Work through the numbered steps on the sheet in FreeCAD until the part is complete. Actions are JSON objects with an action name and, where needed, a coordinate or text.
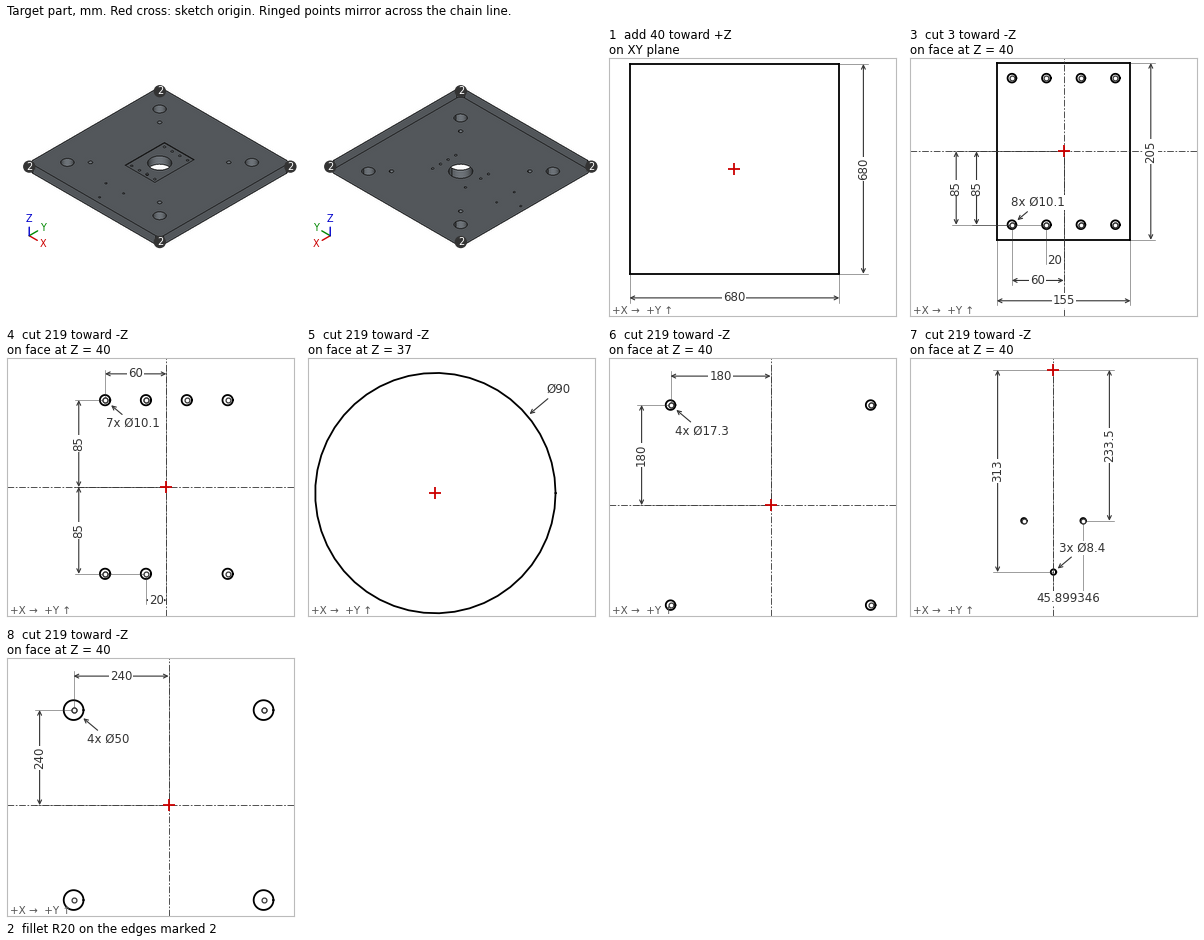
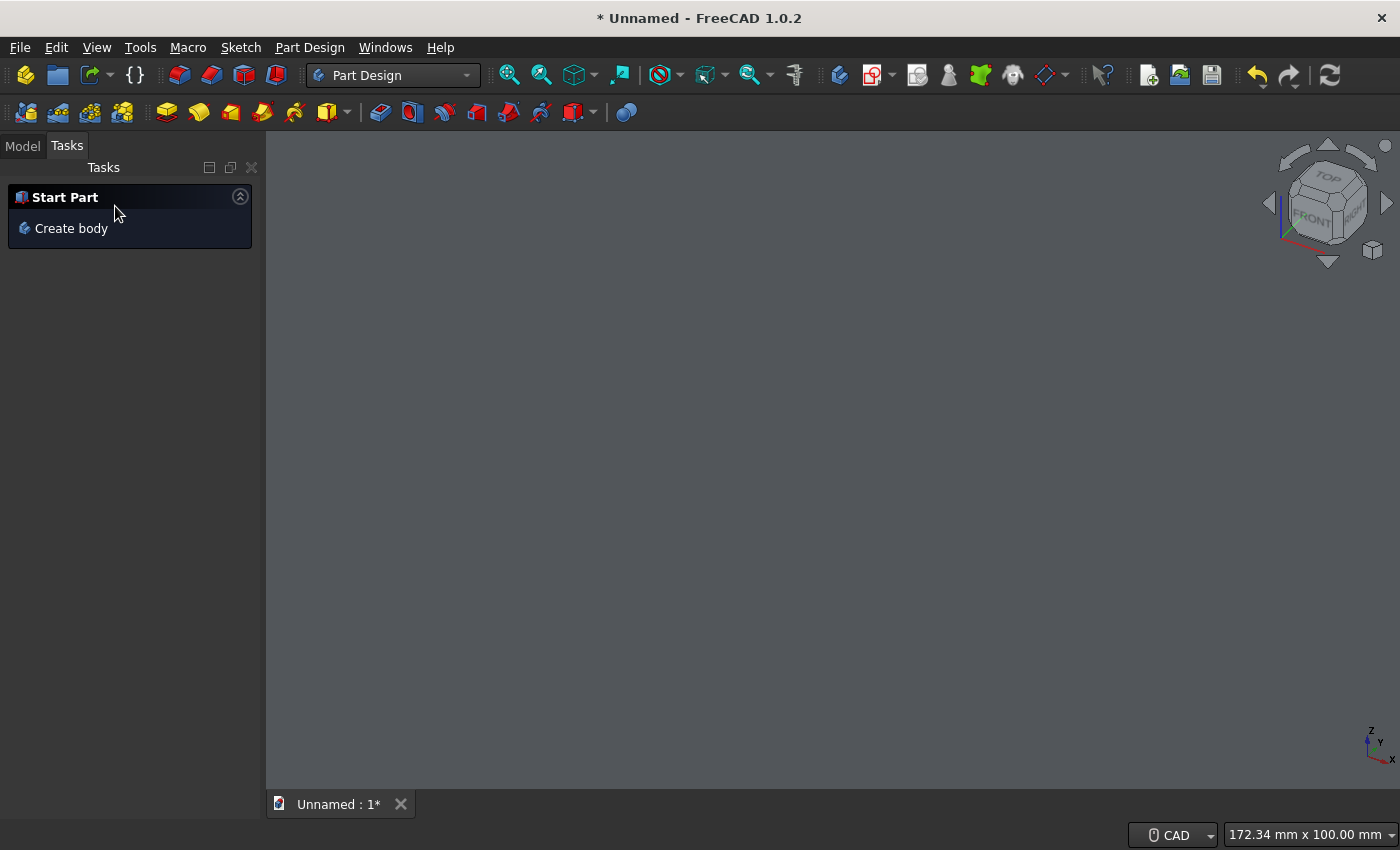
{"action": "left_click", "coordinate": [510, 76]}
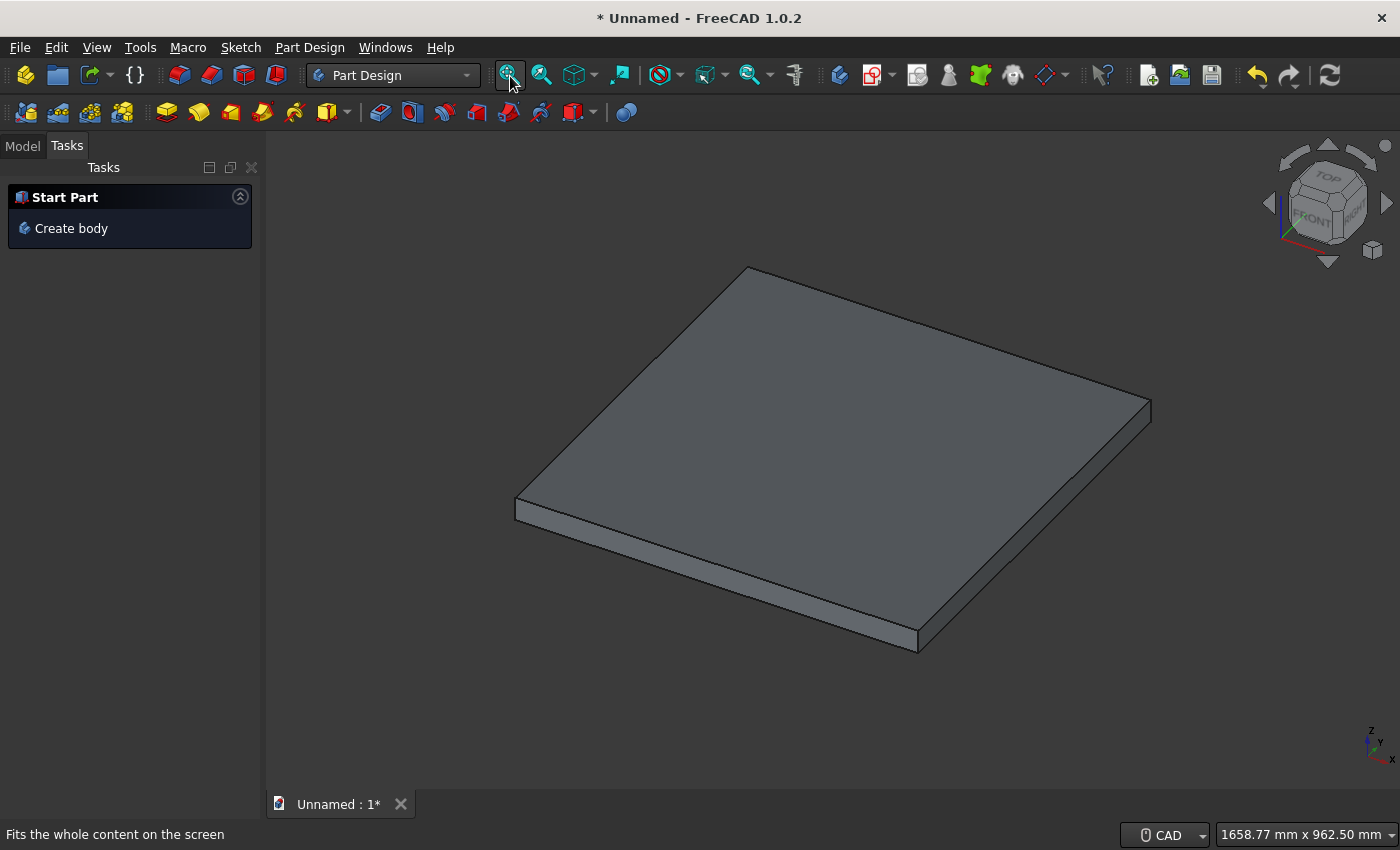
{"action": "left_click", "coordinate": [918, 641]}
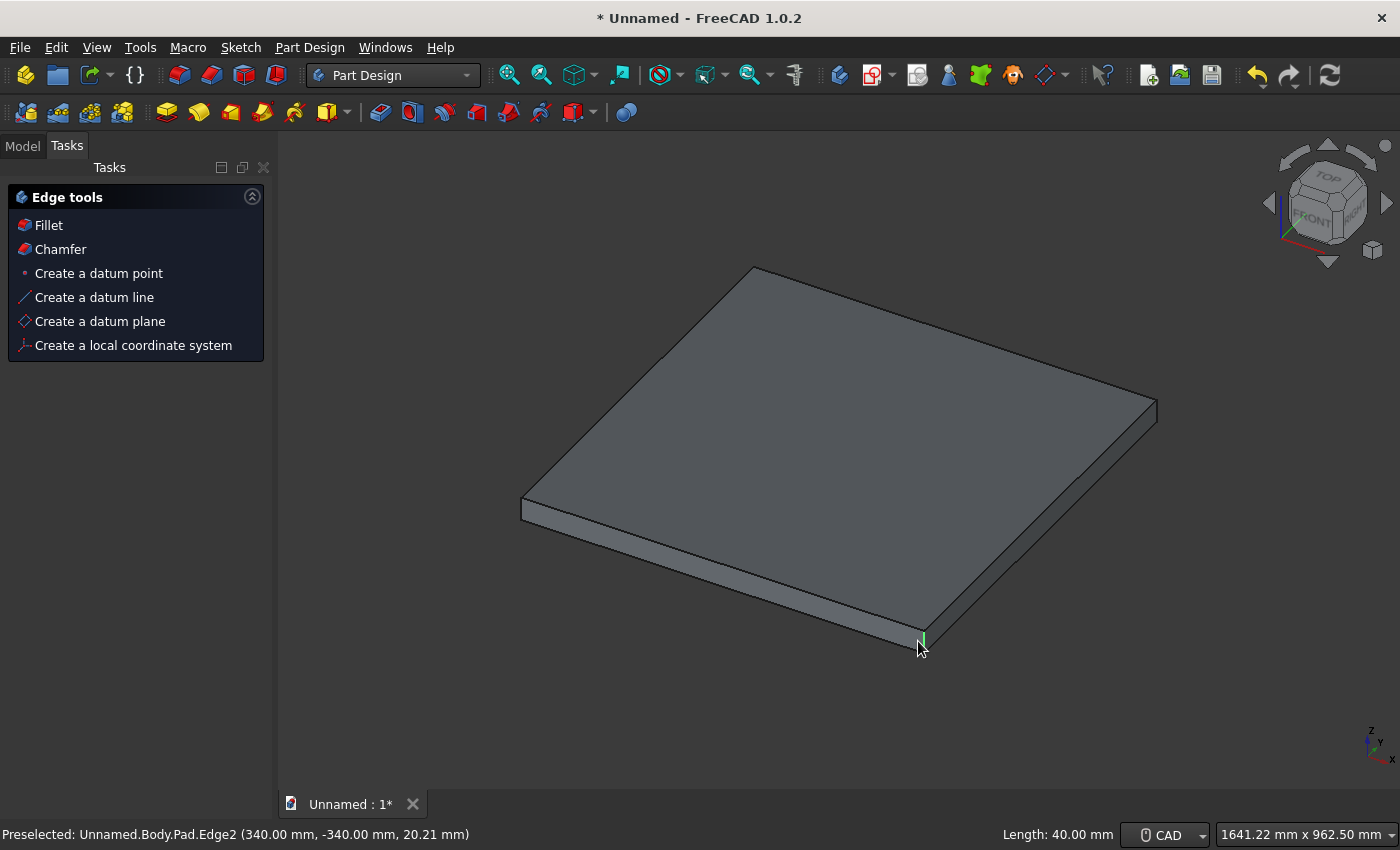
{"action": "key", "text": "0"}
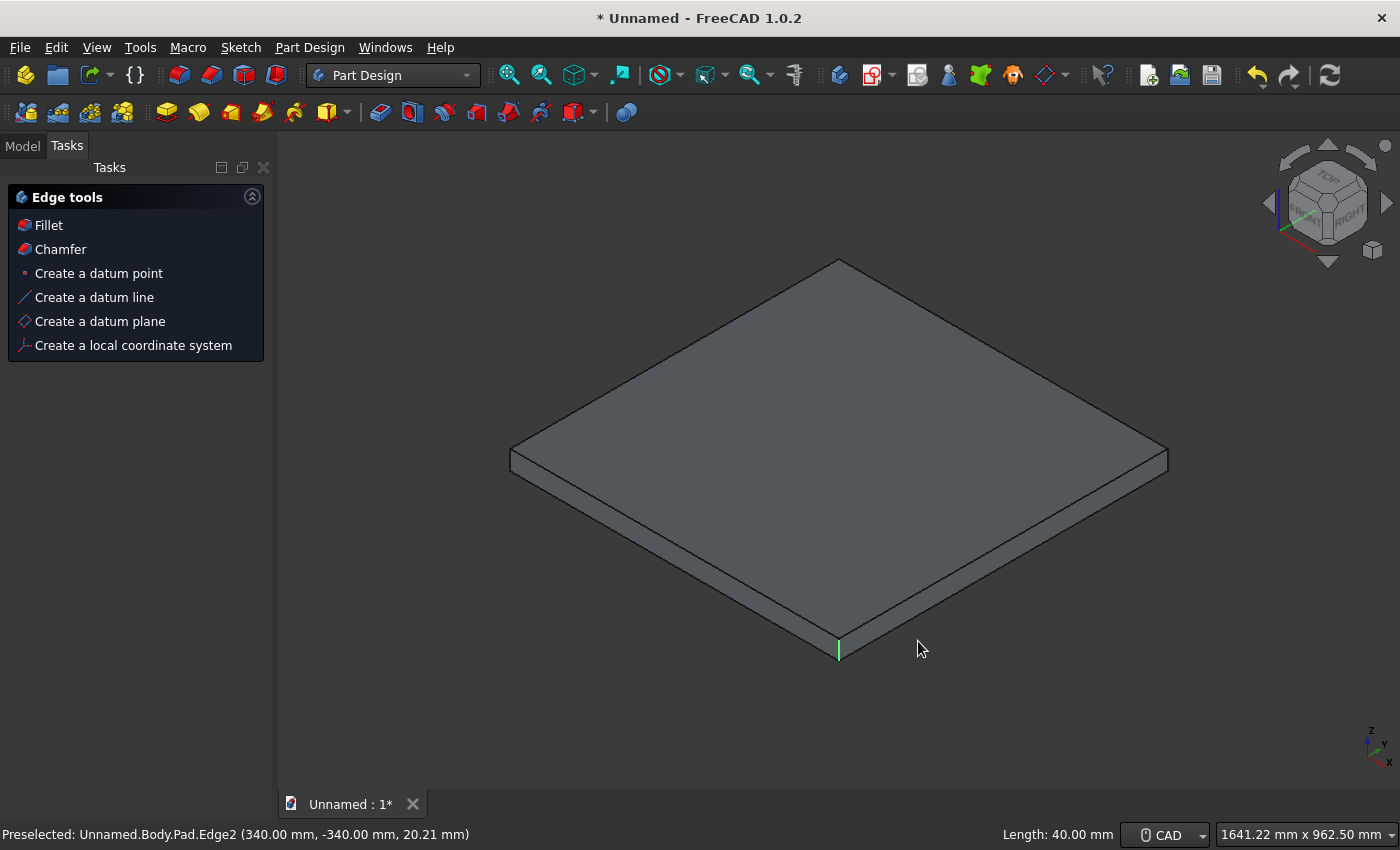
{"action": "key", "text": "2"}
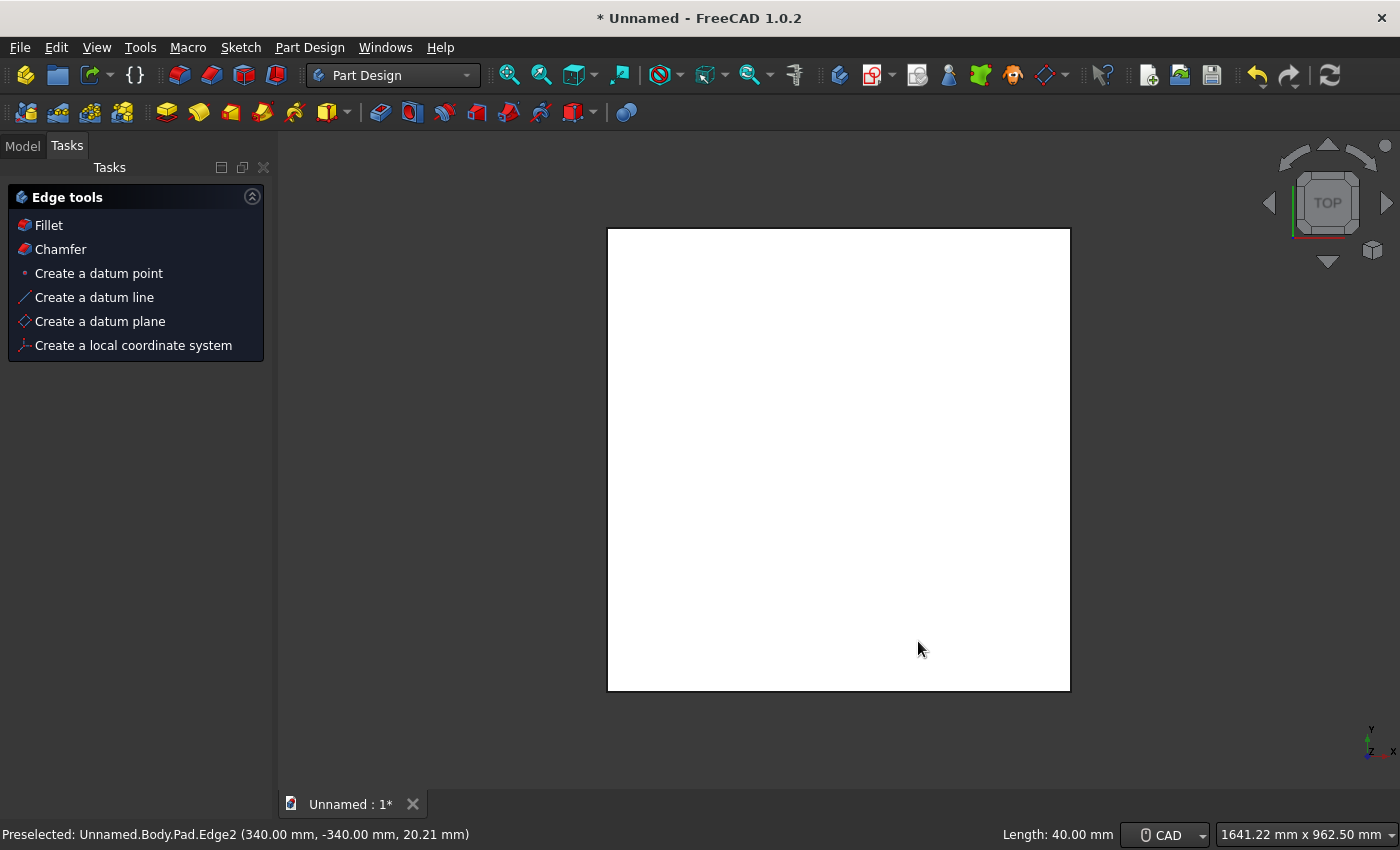
{"action": "key", "text": "1"}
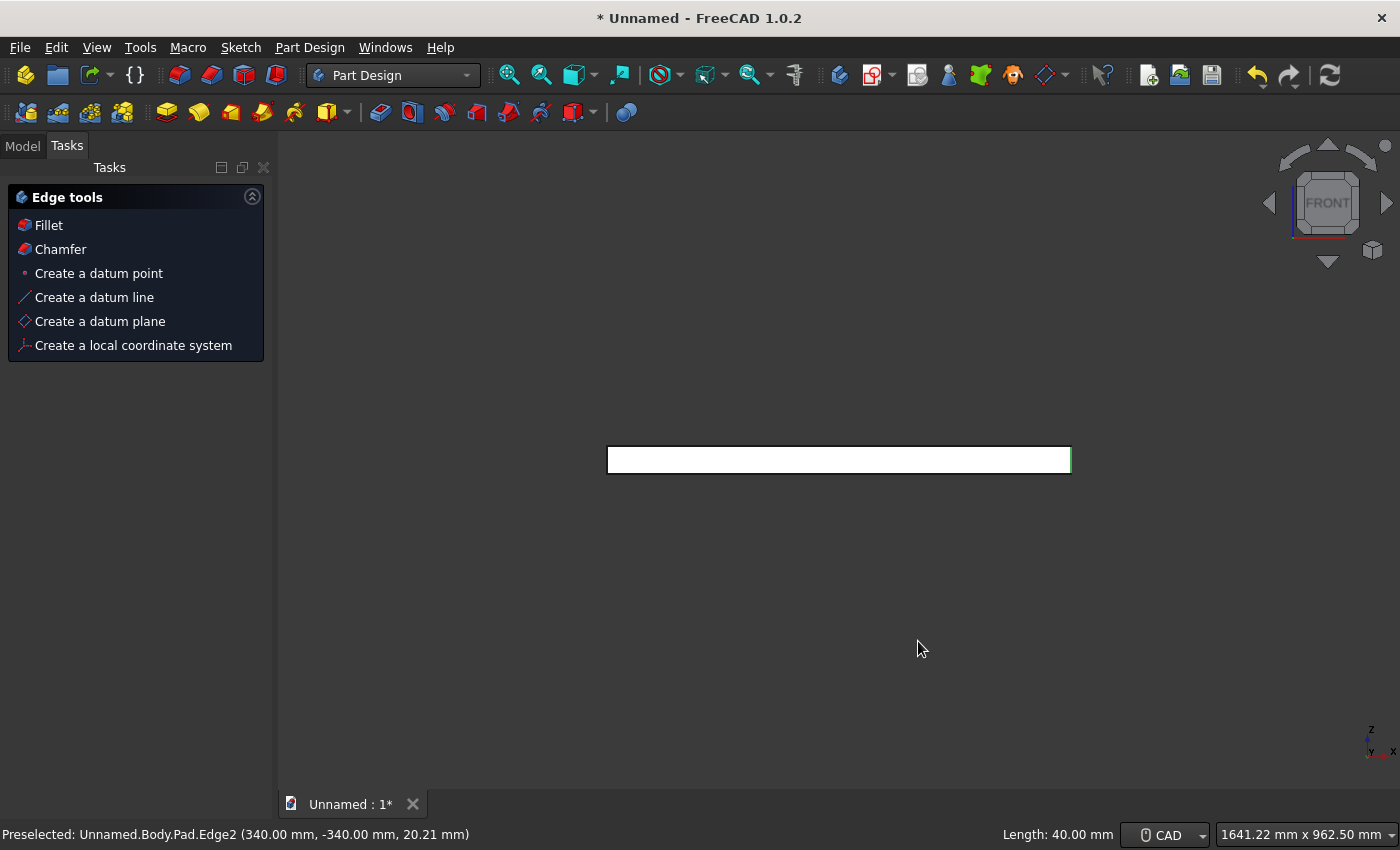
{"action": "left_click", "coordinate": [510, 76]}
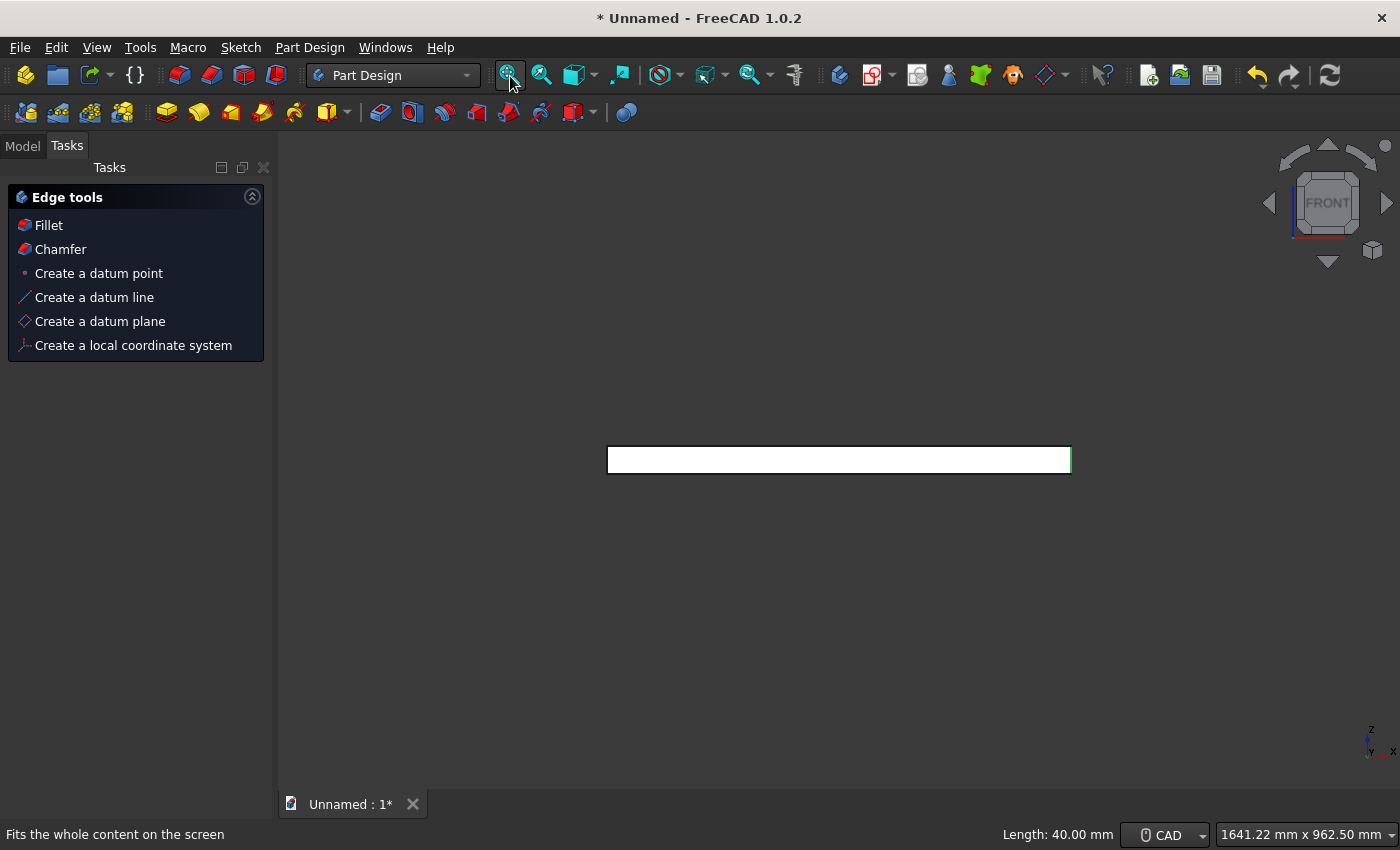
{"action": "left_click", "coordinate": [607, 459], "text": "ctrl"}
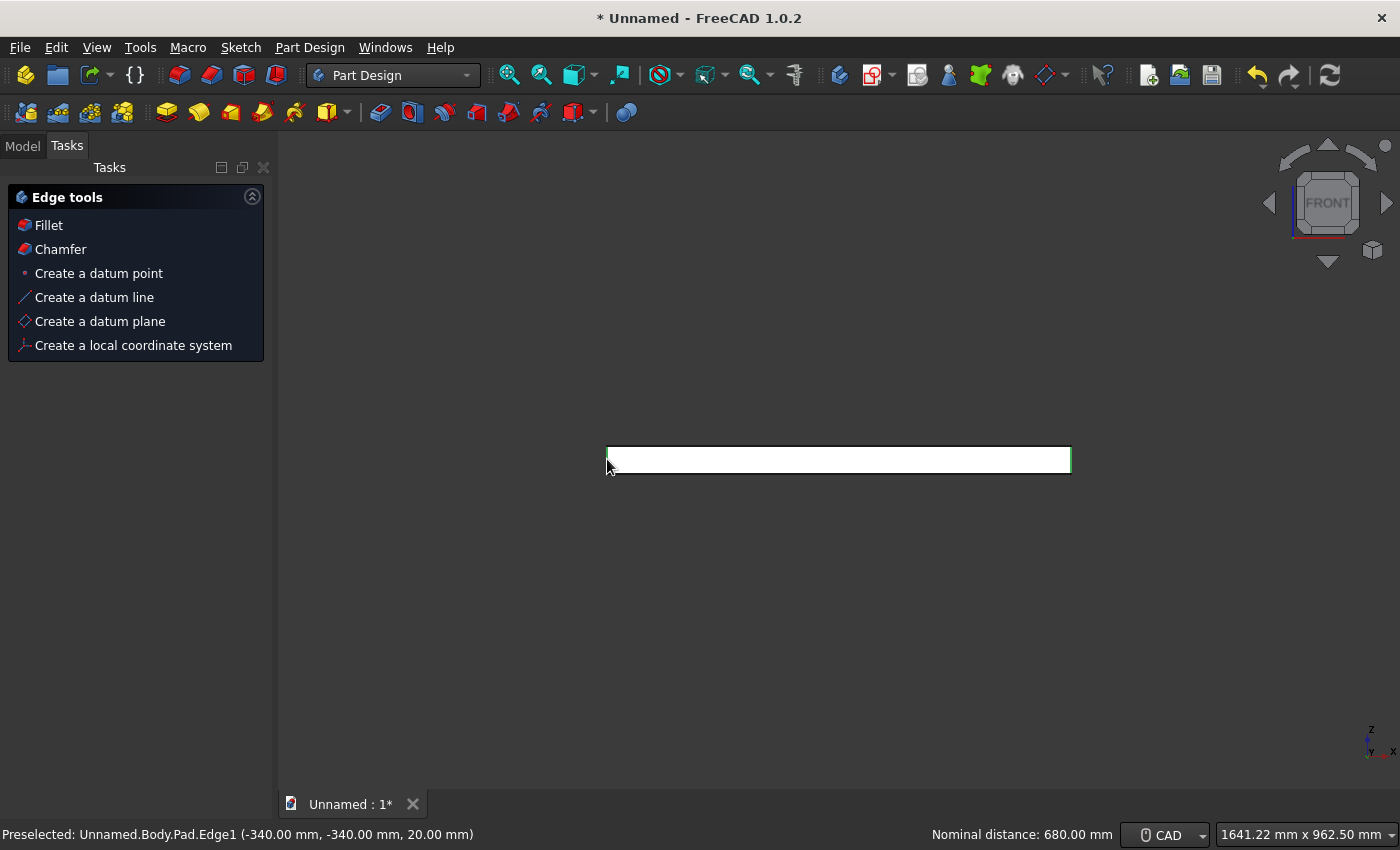
{"action": "key", "text": "3"}